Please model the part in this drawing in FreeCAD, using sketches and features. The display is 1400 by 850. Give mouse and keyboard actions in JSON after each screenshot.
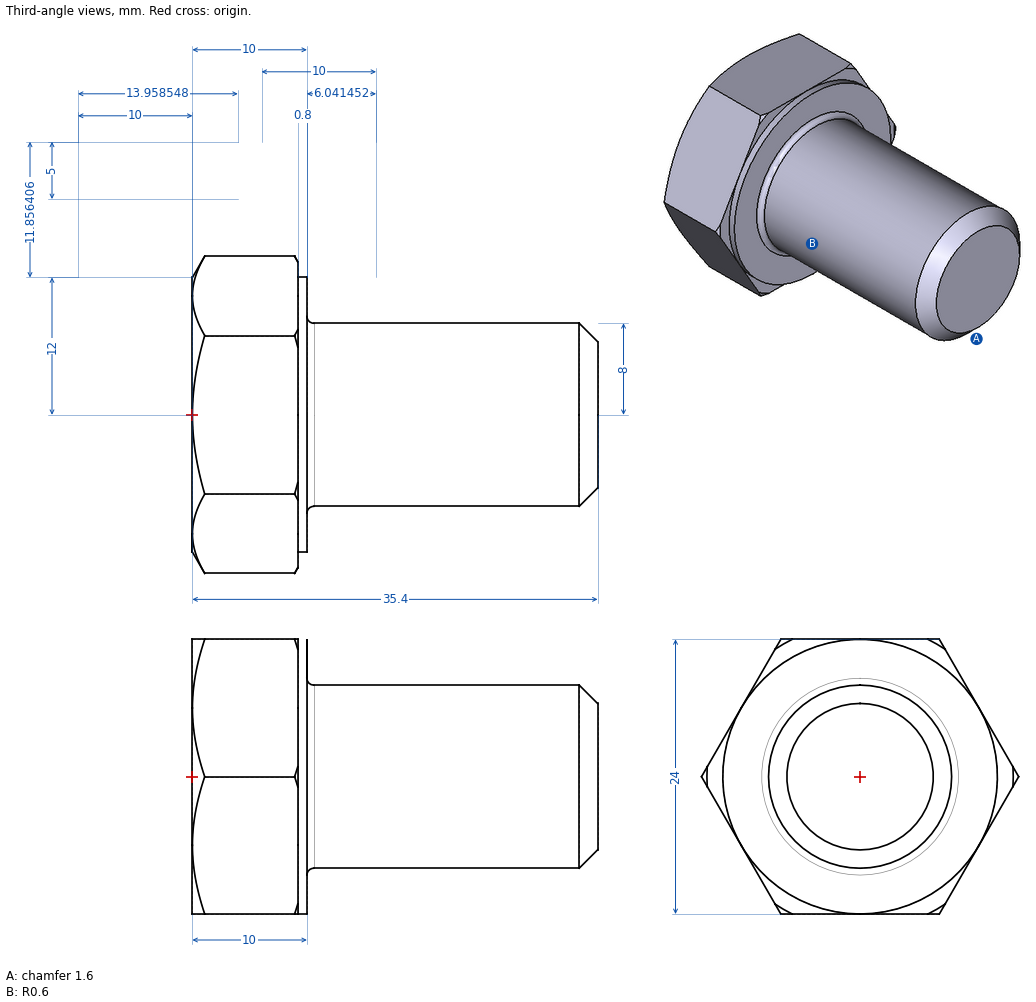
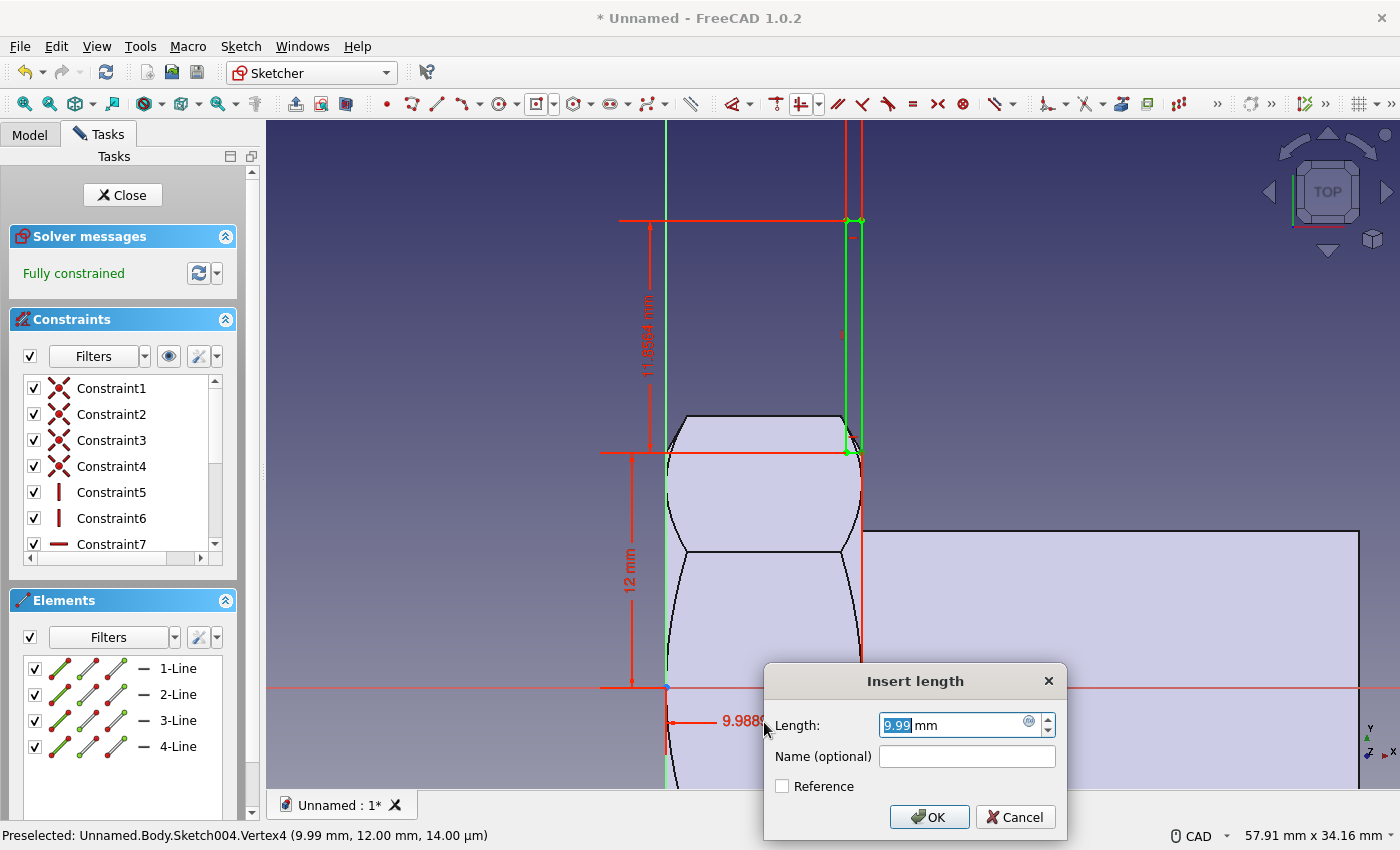
{"action": "type", "text": "10"}
{"action": "key", "text": "Return"}
{"action": "key", "text": "Escape"}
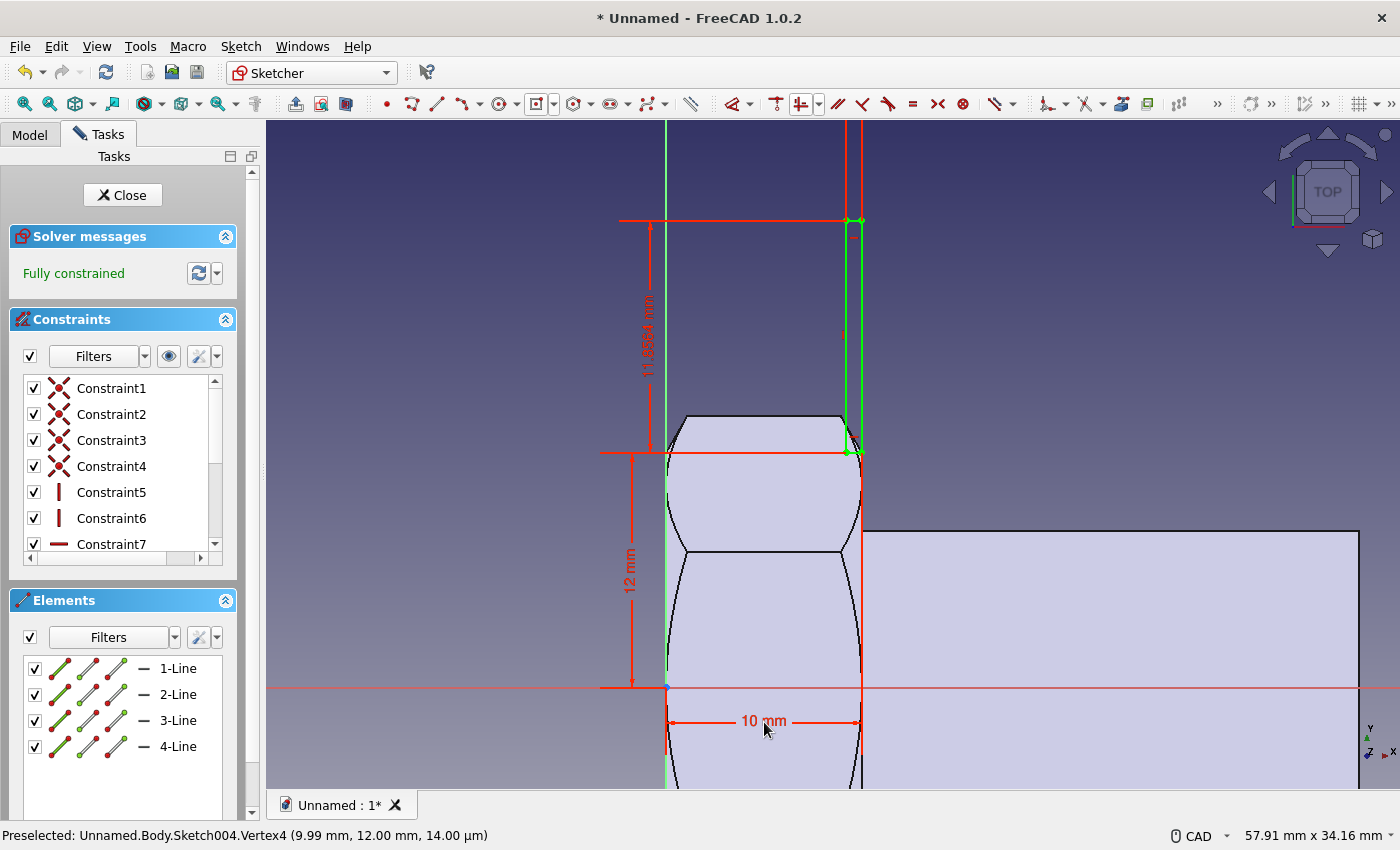
{"action": "left_click", "coordinate": [123, 195]}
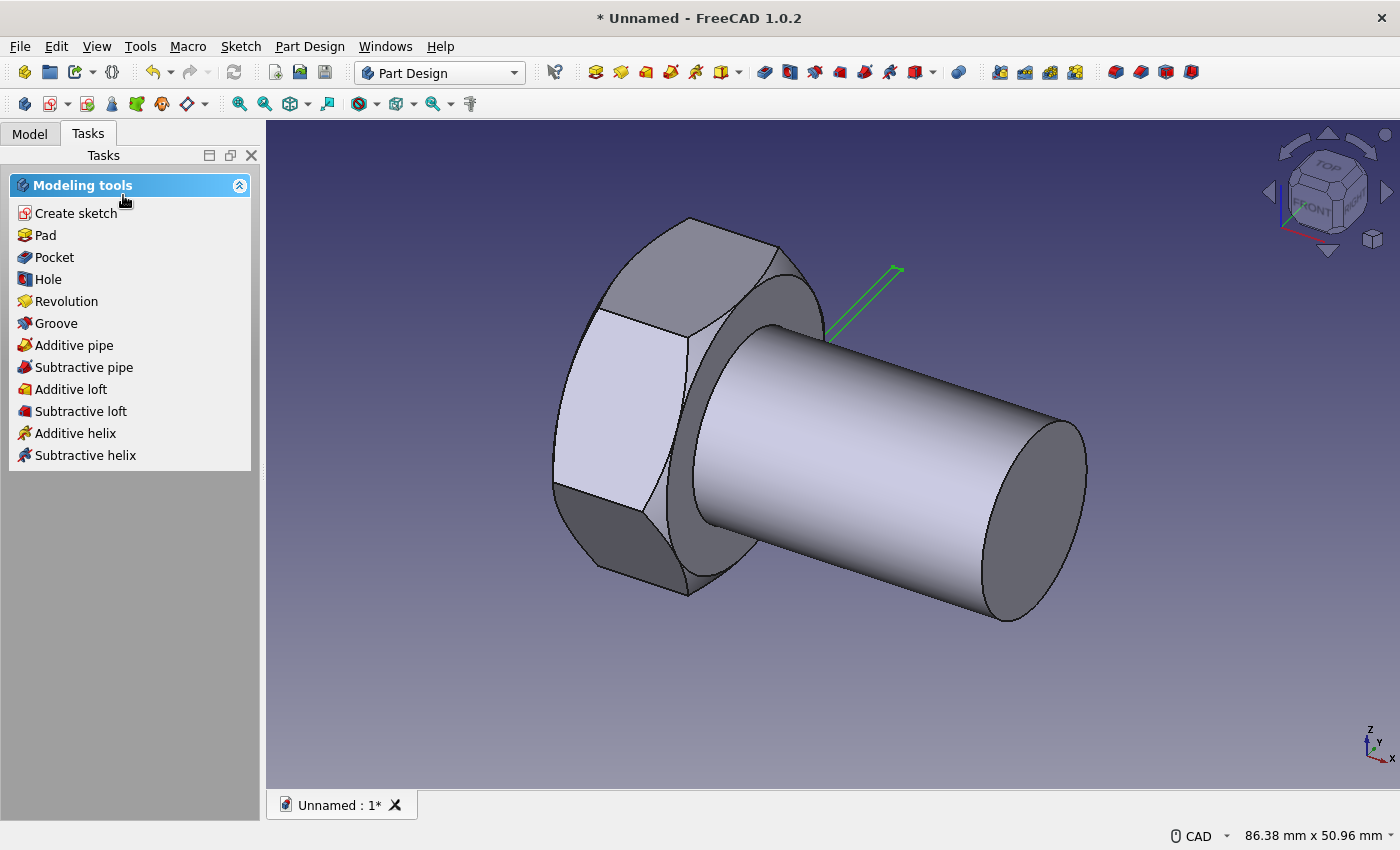
{"action": "left_click", "coordinate": [815, 72]}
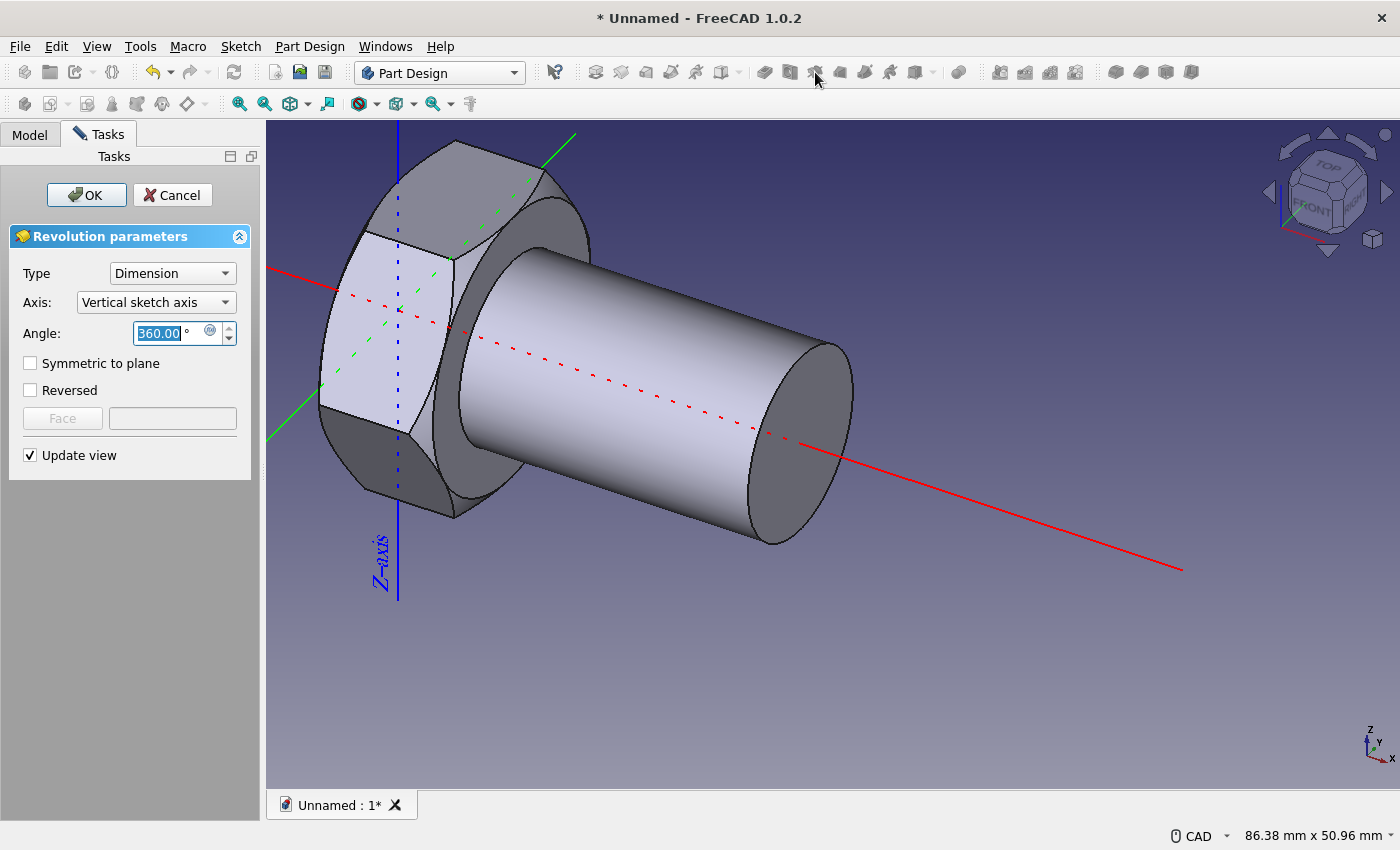
{"action": "left_click", "coordinate": [157, 302]}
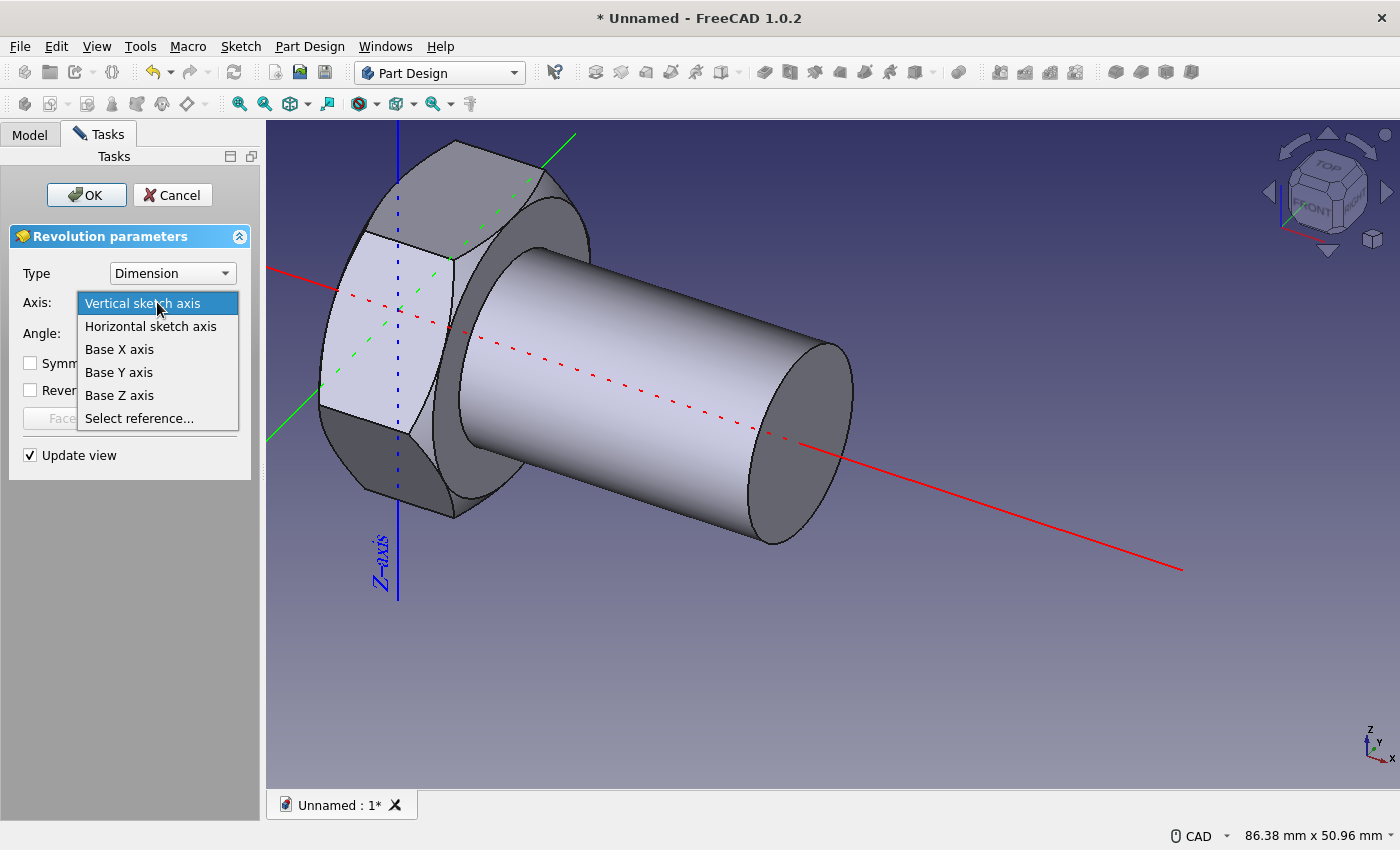
{"action": "left_click", "coordinate": [156, 326]}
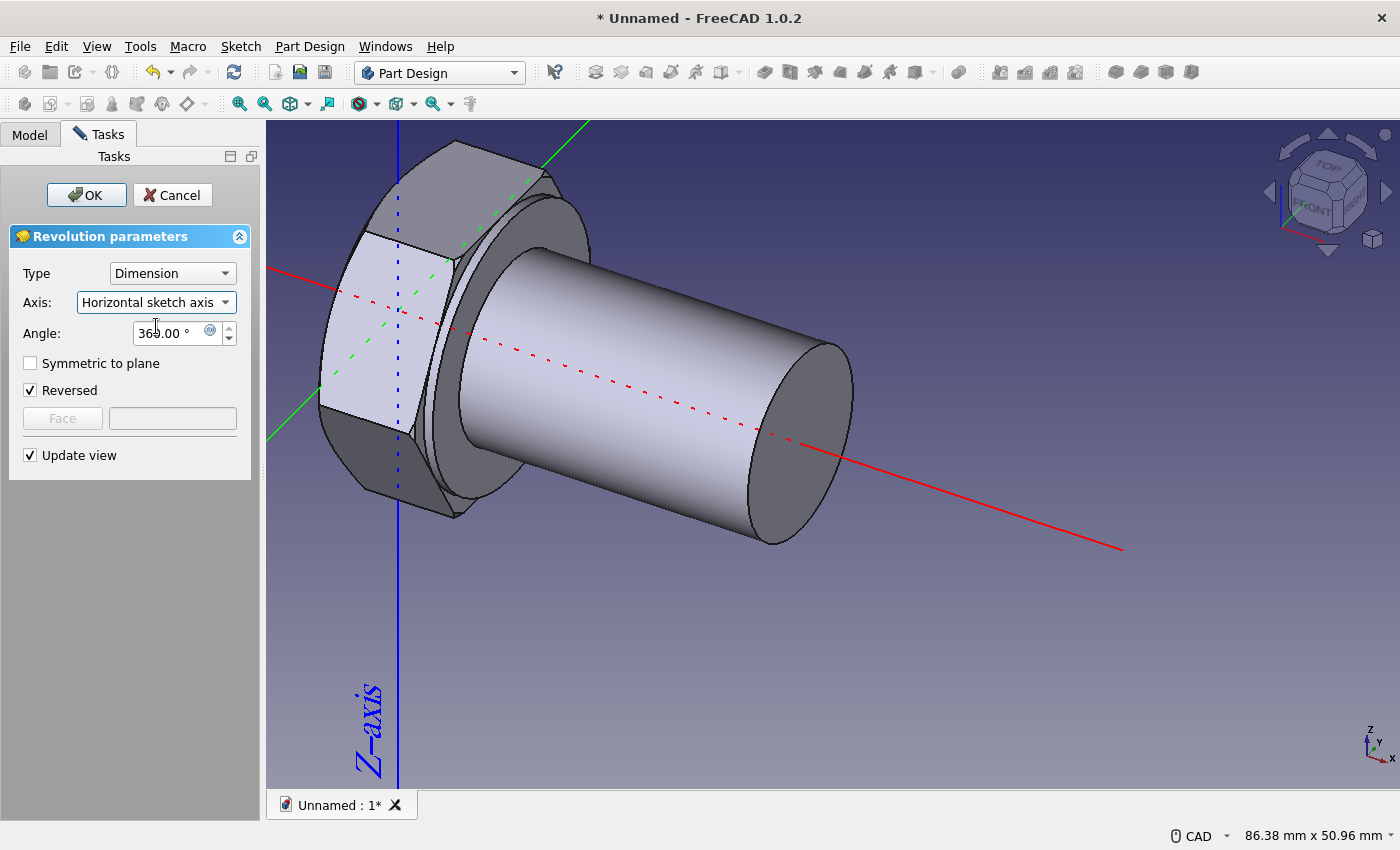
{"action": "left_click", "coordinate": [87, 195]}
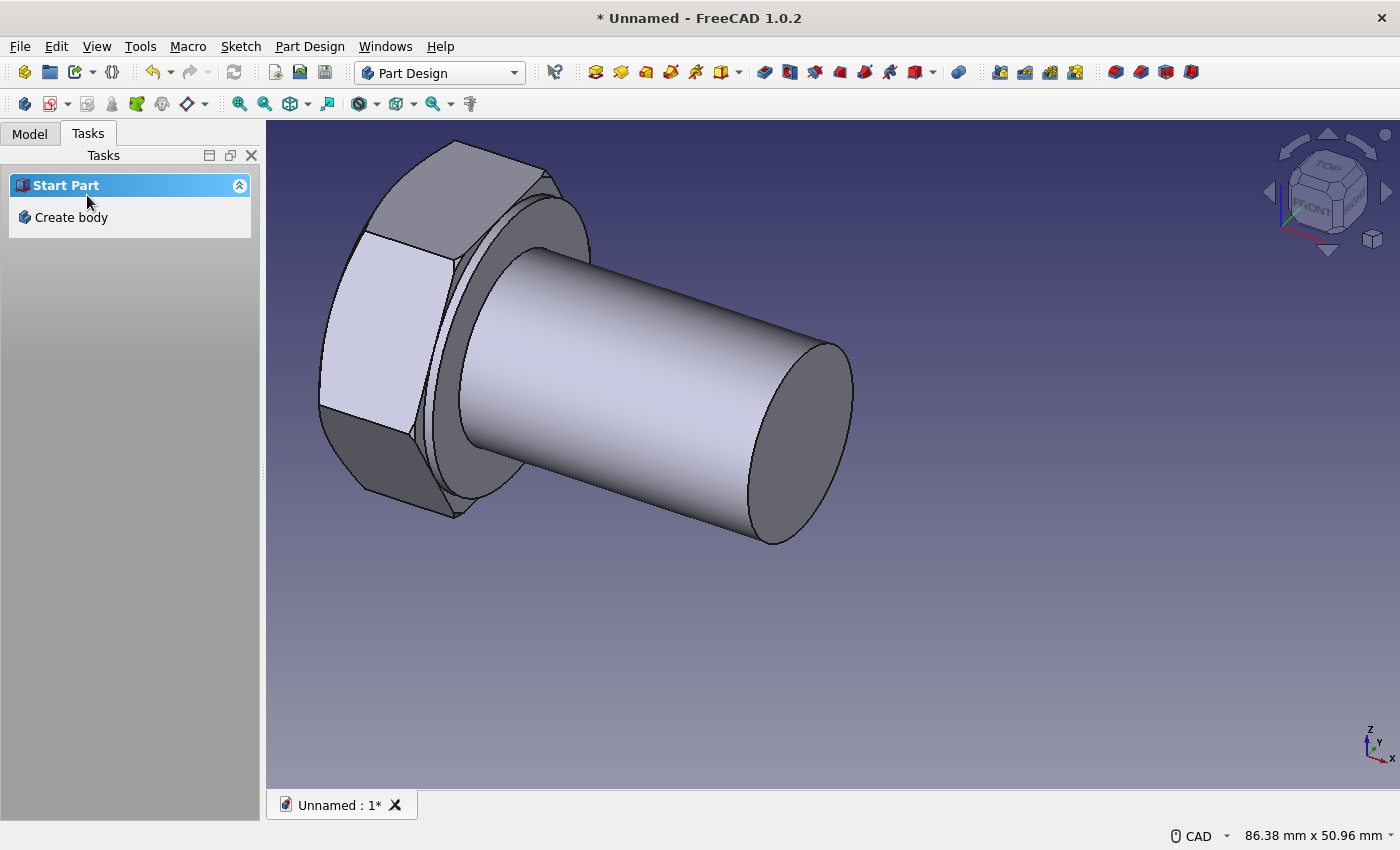
{"action": "key", "text": "v f"}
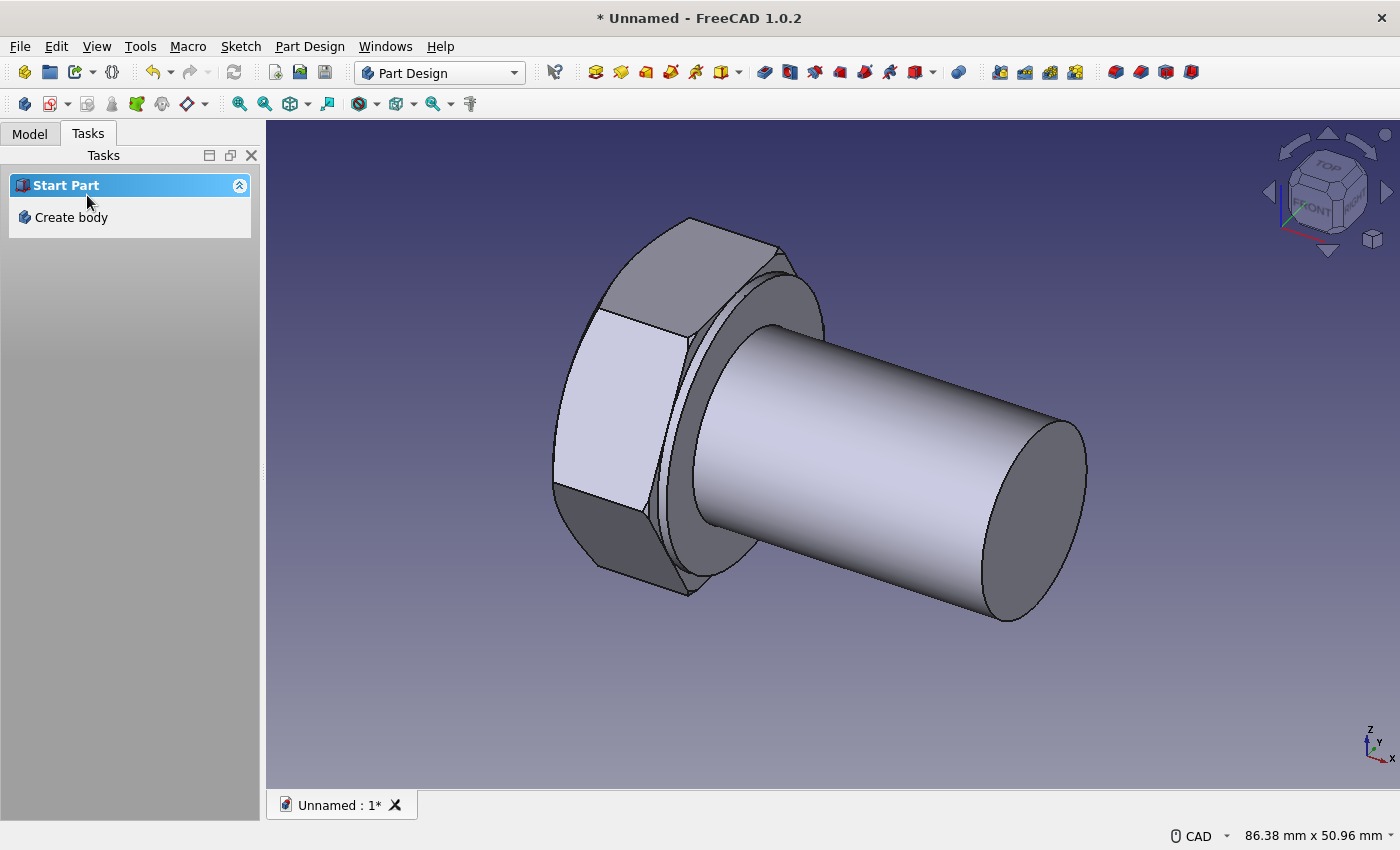
{"action": "left_click", "coordinate": [982, 572]}